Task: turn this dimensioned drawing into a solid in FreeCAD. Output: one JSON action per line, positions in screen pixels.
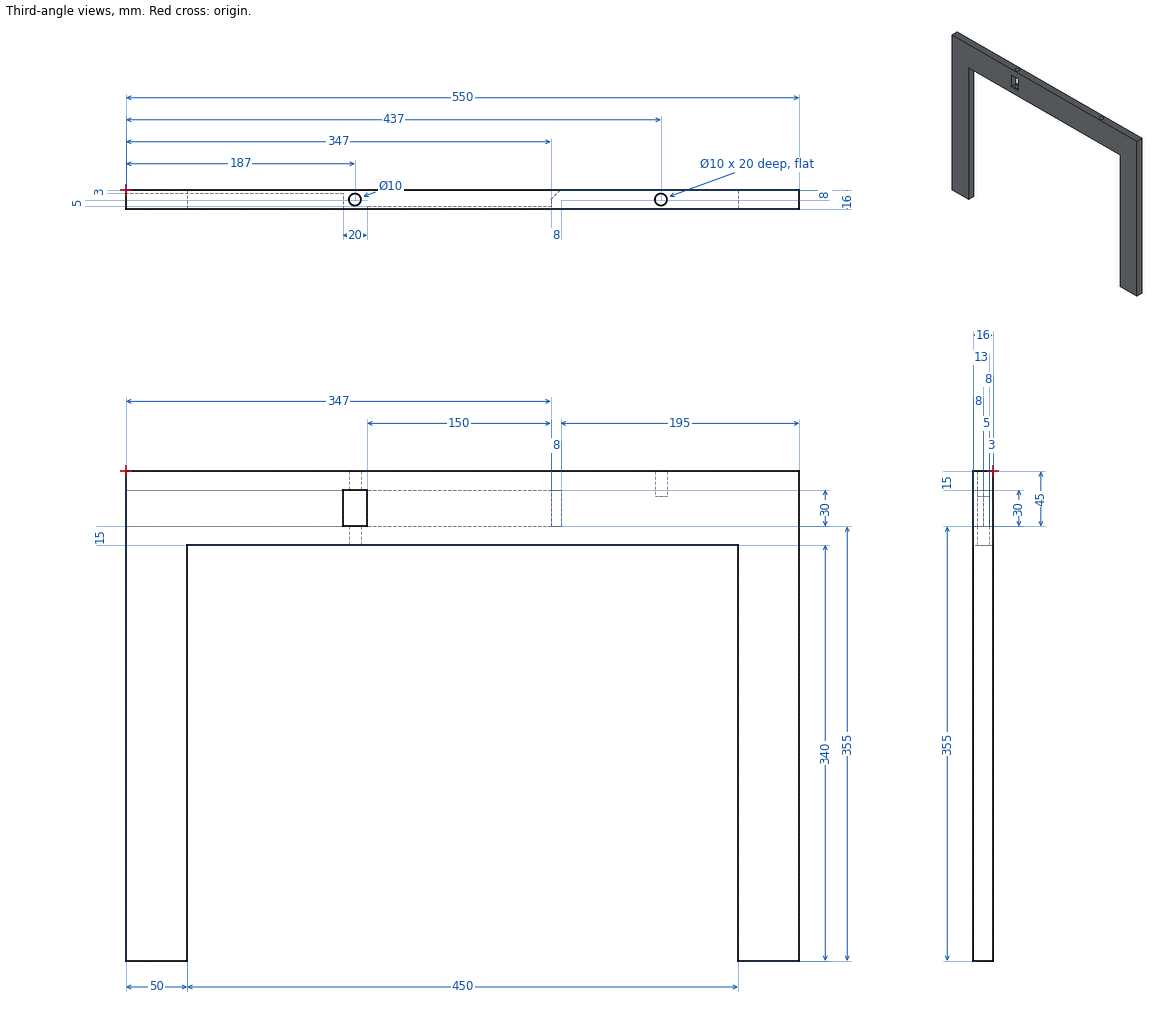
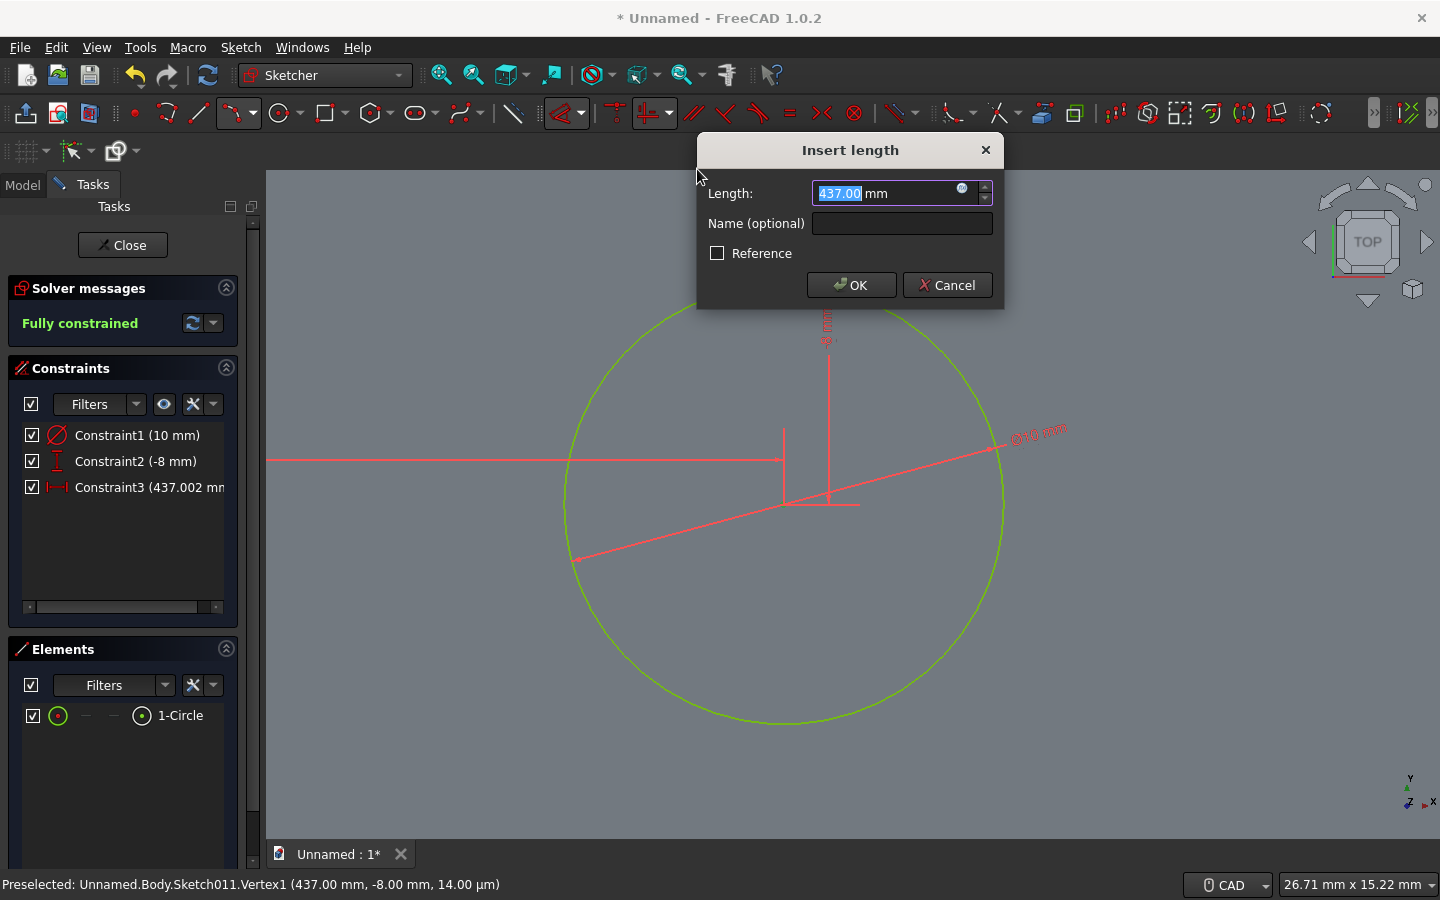
{"action": "type", "text": "437"}
{"action": "key", "text": "Return"}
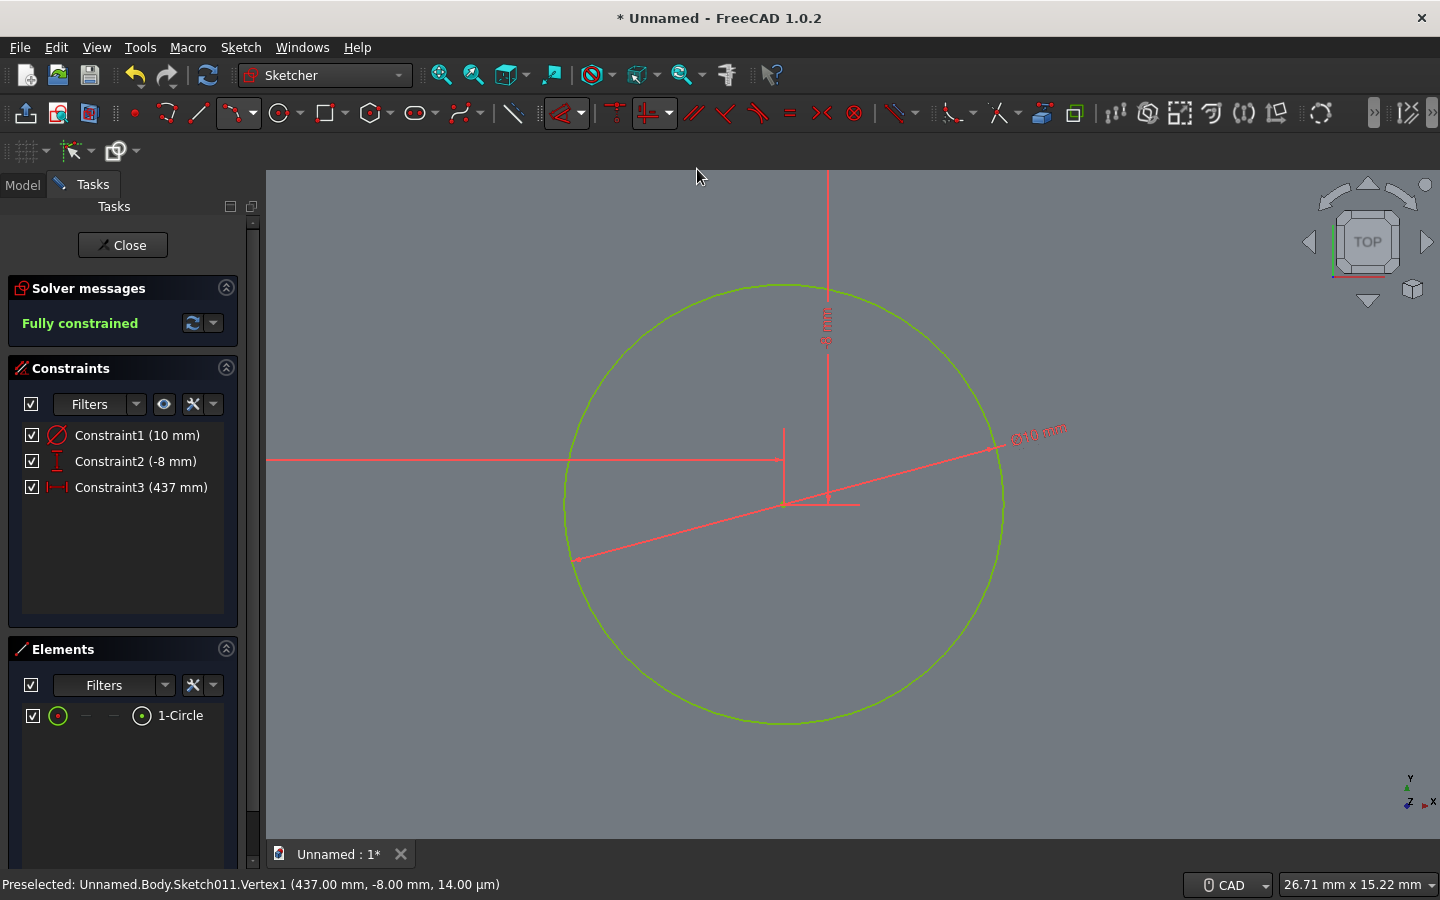
{"action": "left_click", "coordinate": [123, 245]}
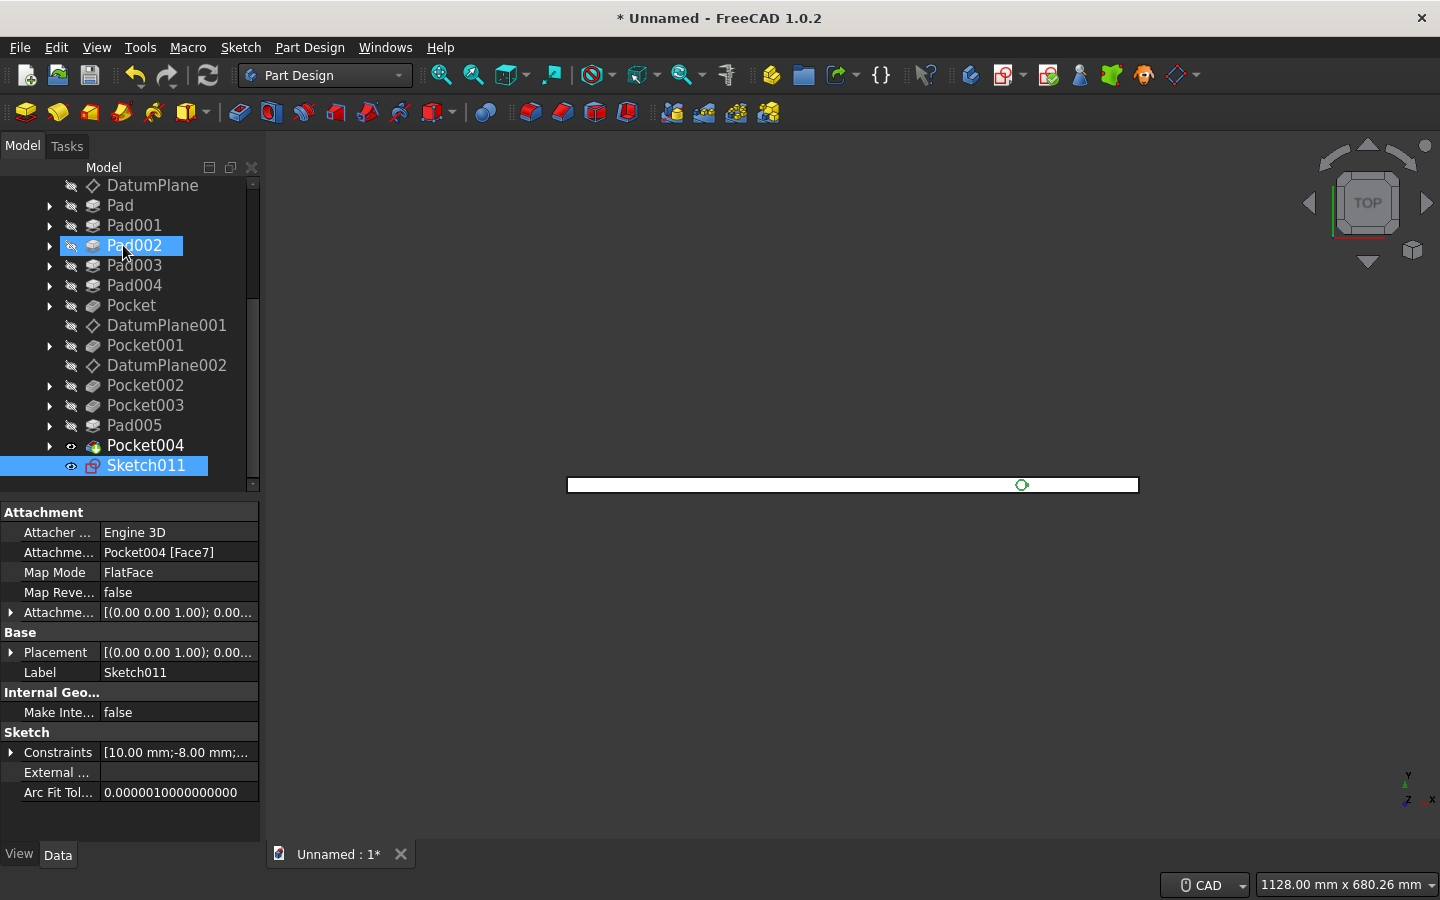
{"action": "left_click", "coordinate": [272, 112]}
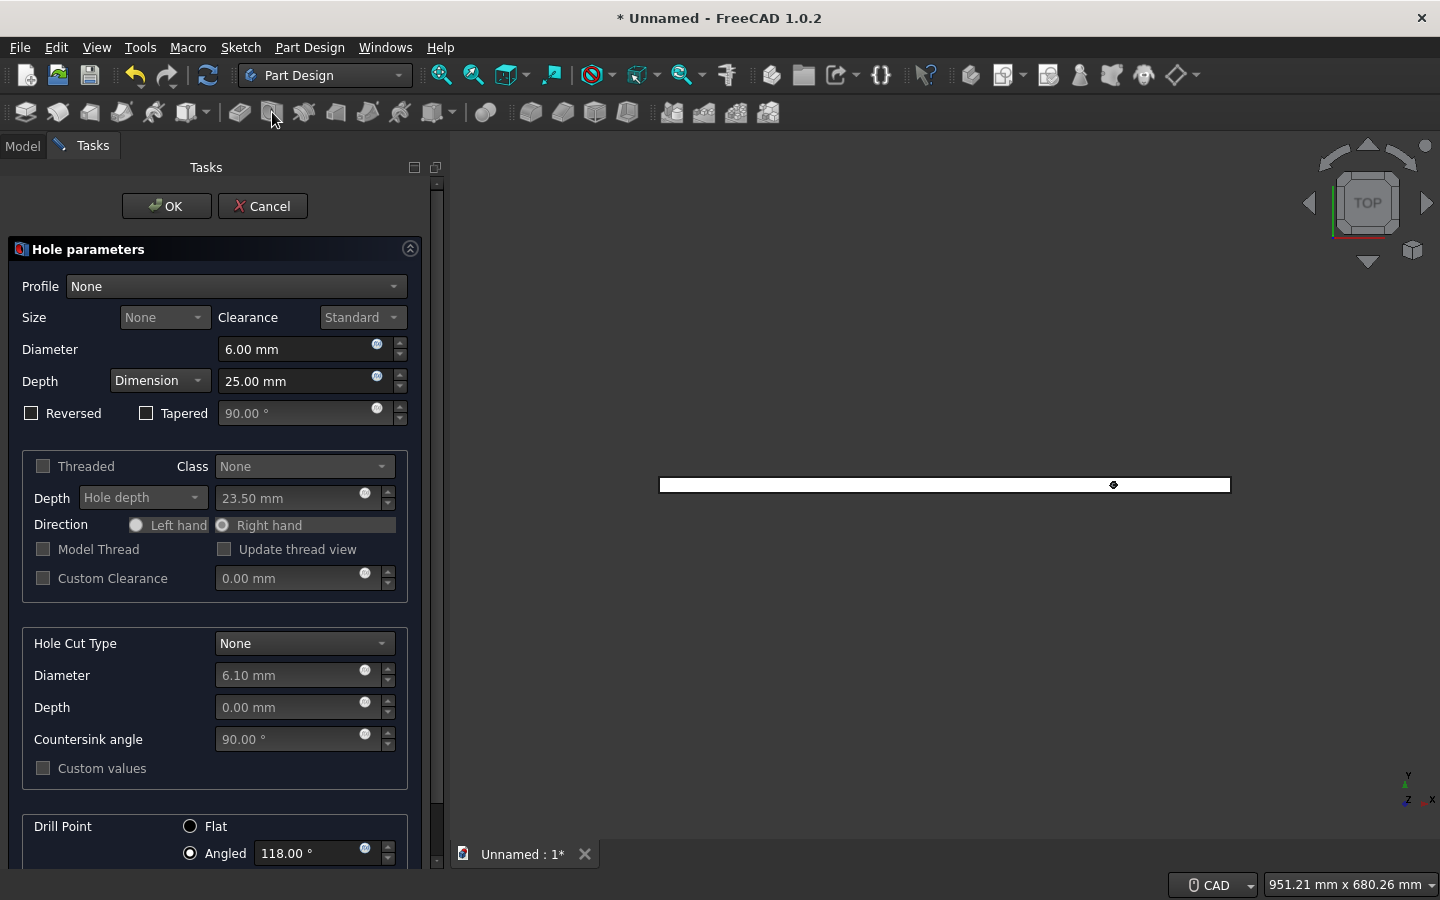
{"action": "triple_click", "coordinate": [305, 349]}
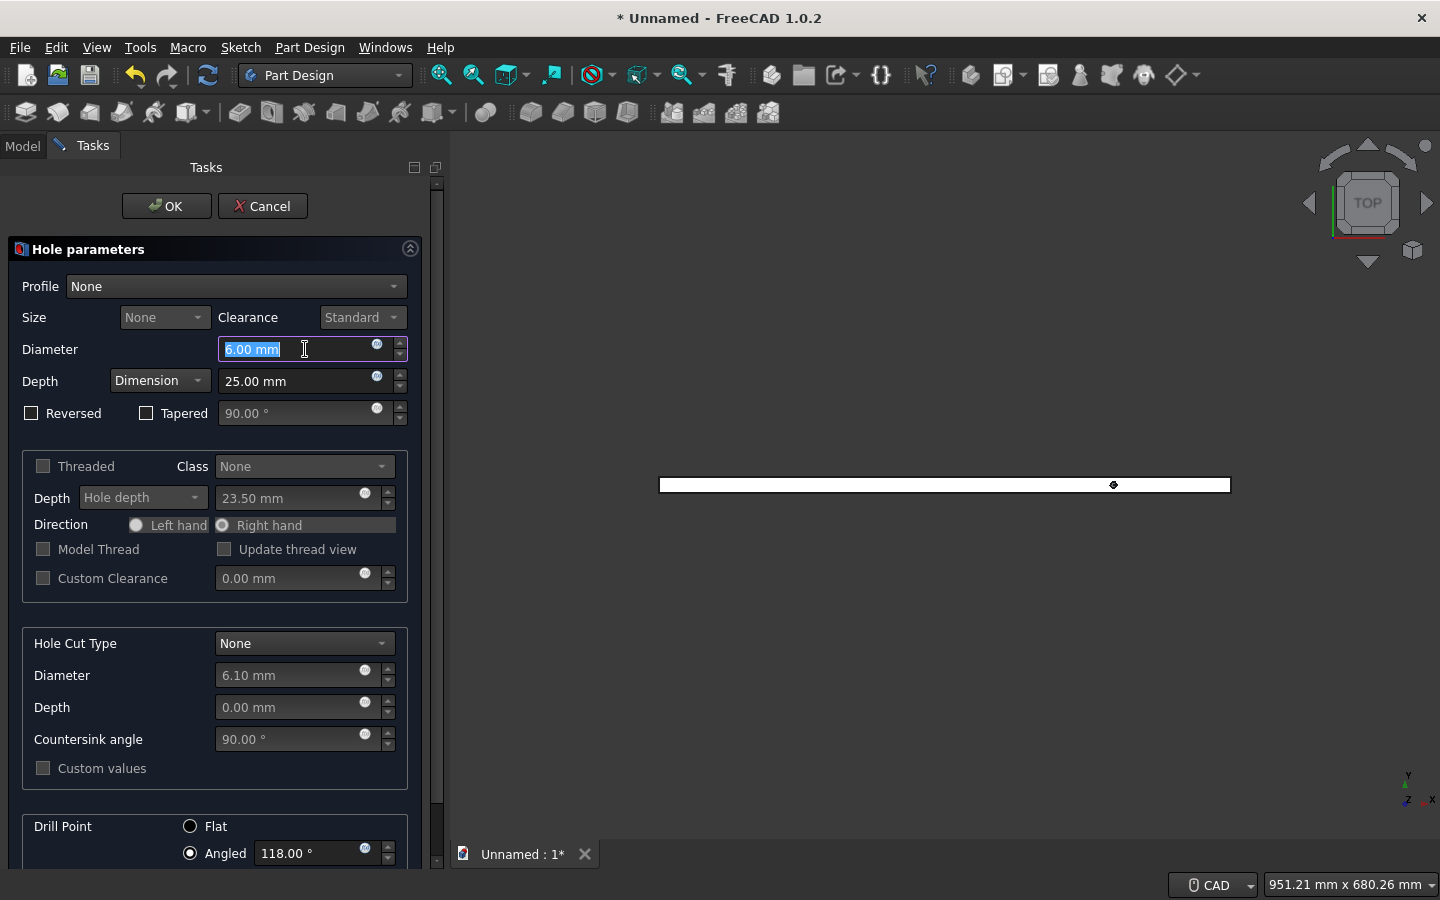
{"action": "type", "text": "10"}
{"action": "key", "text": "Tab"}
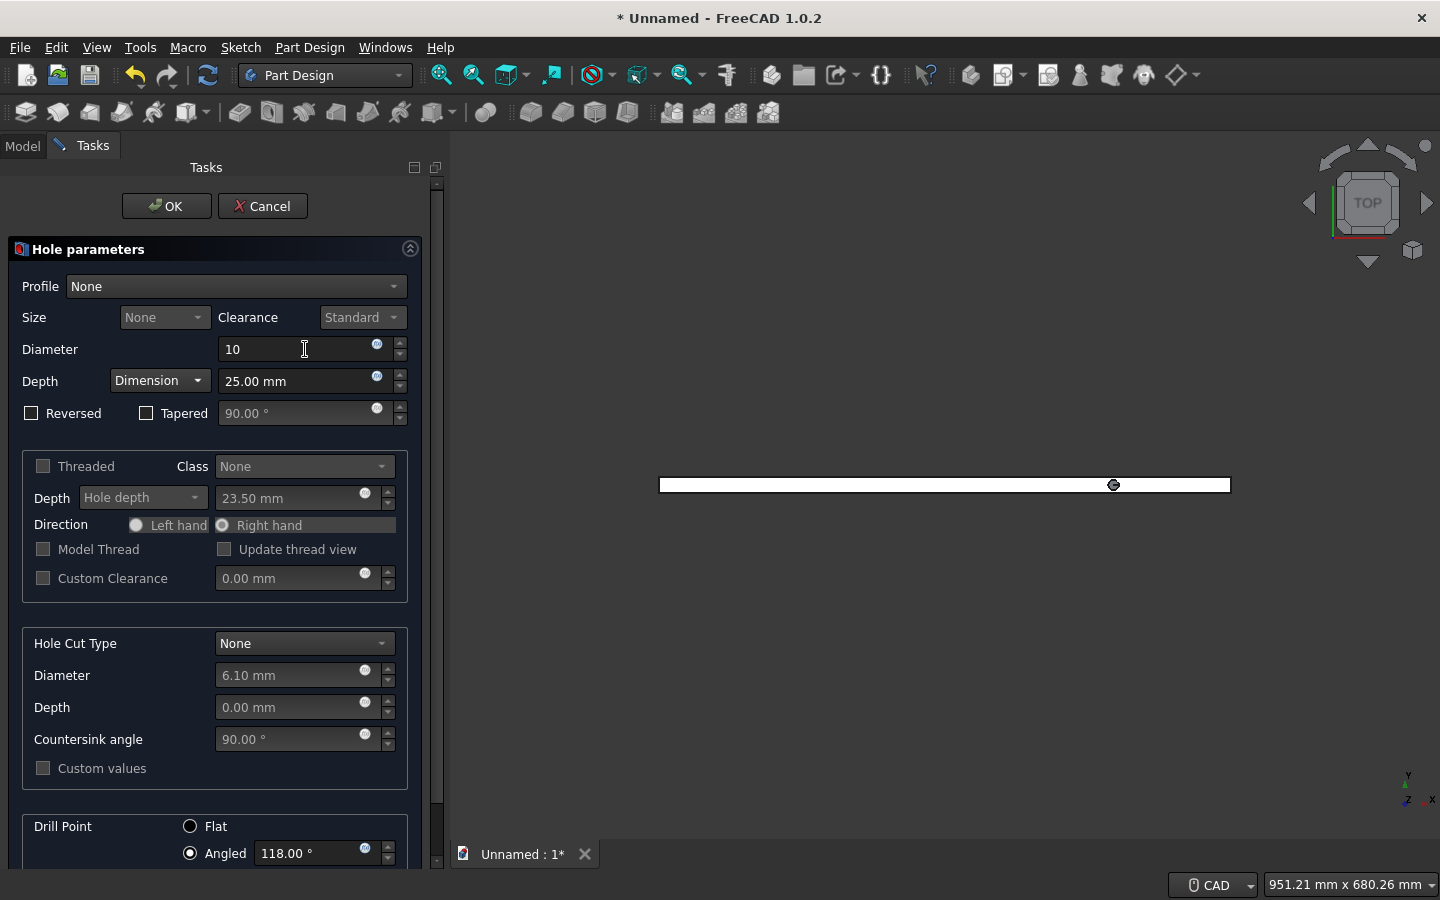
{"action": "triple_click", "coordinate": [305, 381]}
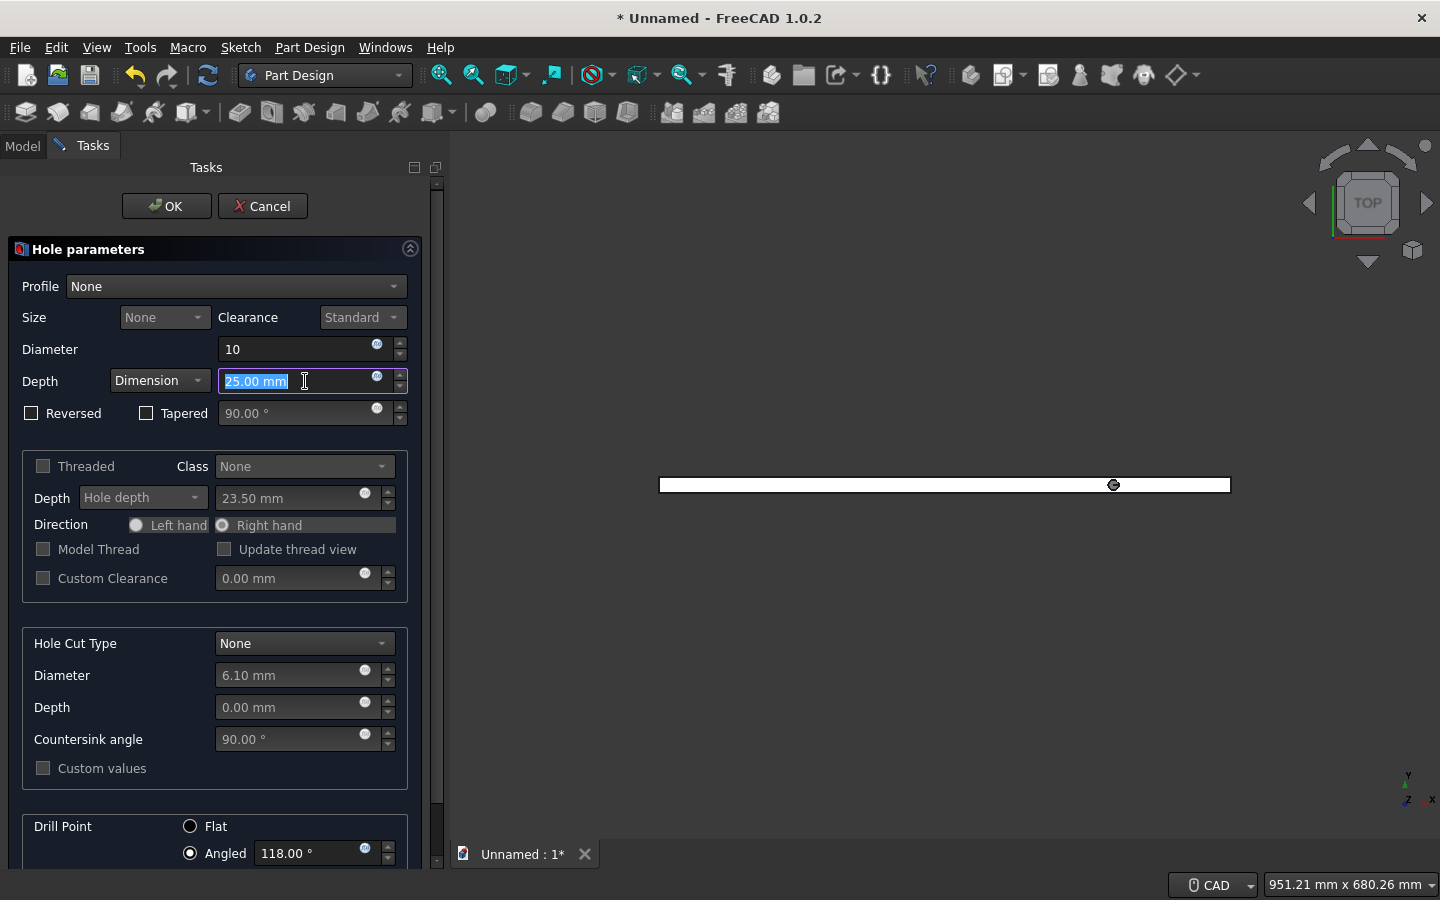
{"action": "type", "text": "20"}
{"action": "key", "text": "Tab"}